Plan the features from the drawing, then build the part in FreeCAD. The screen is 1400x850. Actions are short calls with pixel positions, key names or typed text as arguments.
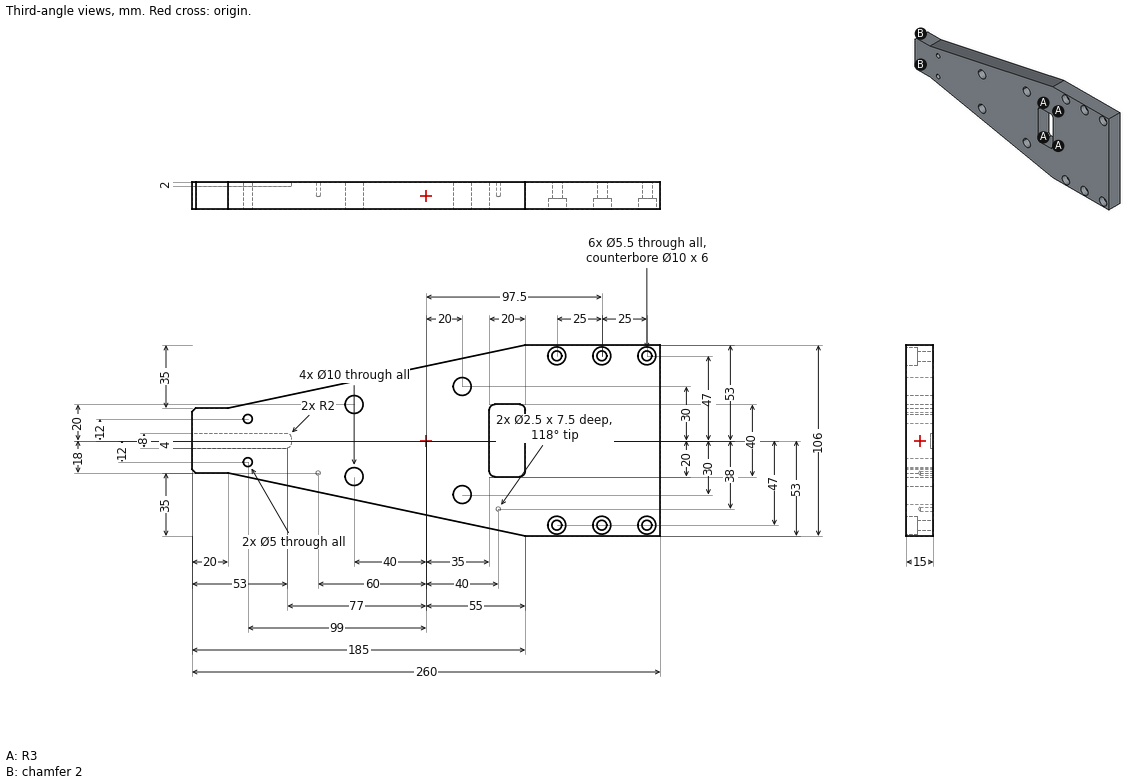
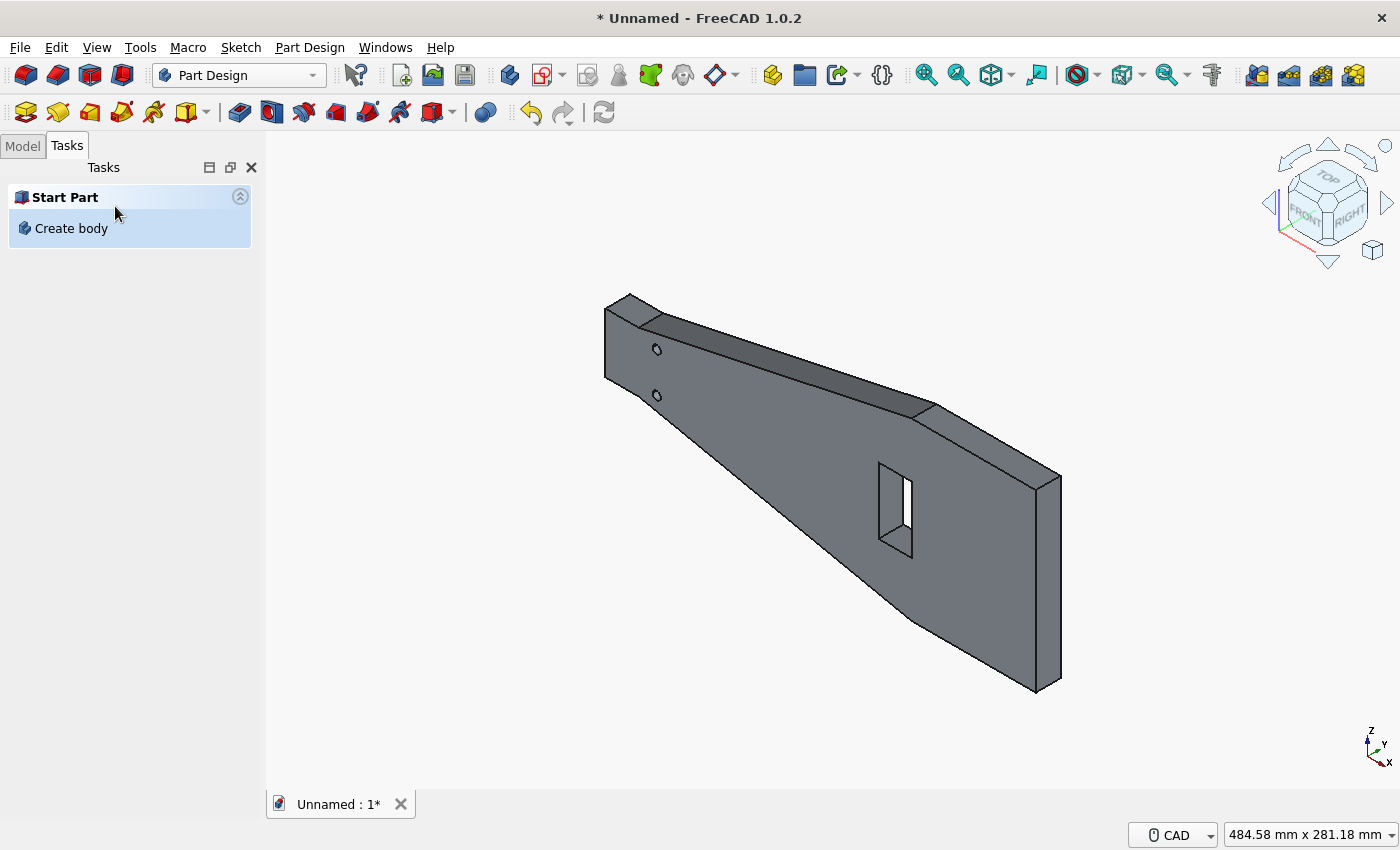
key(2)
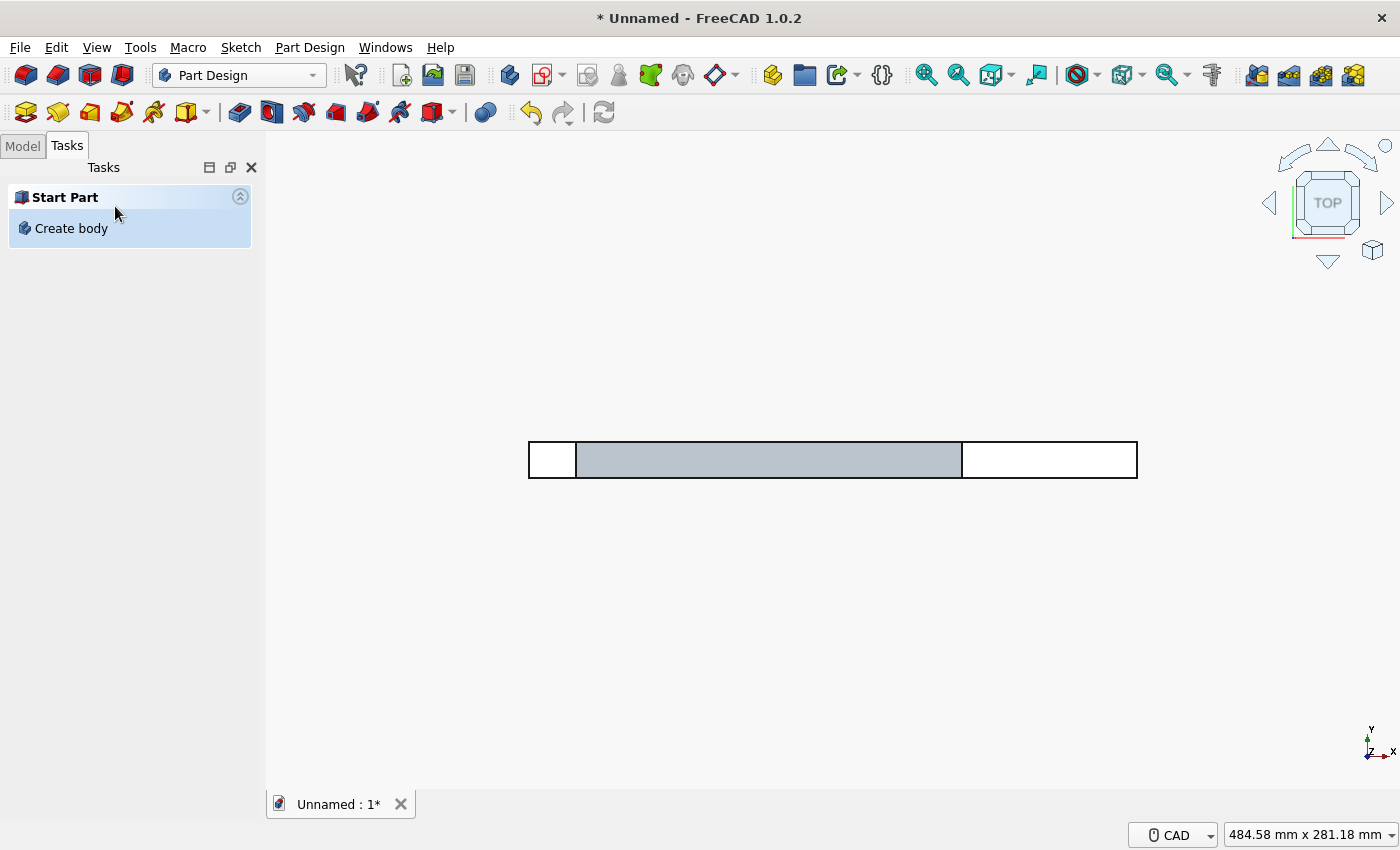
key(1)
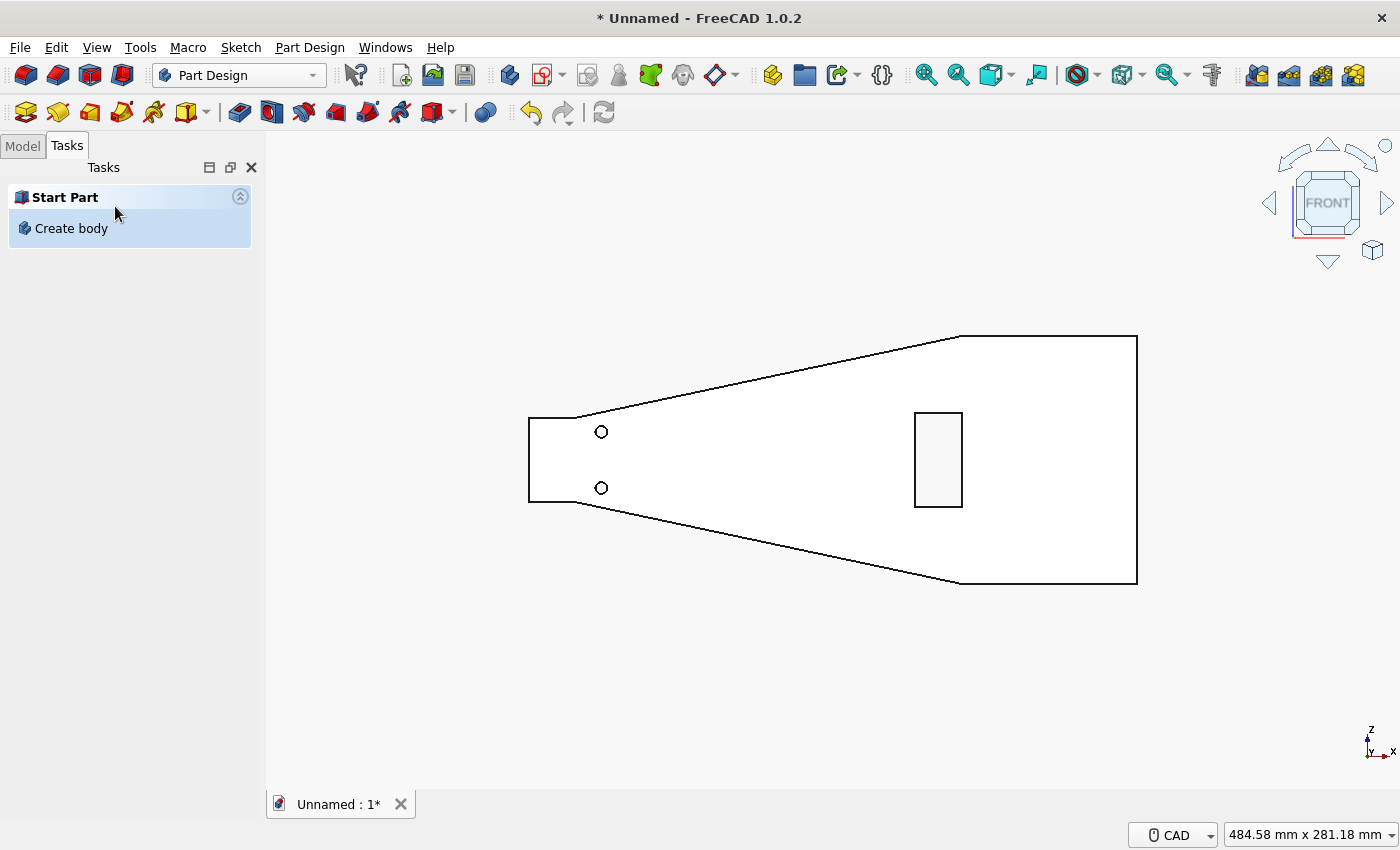
key(3)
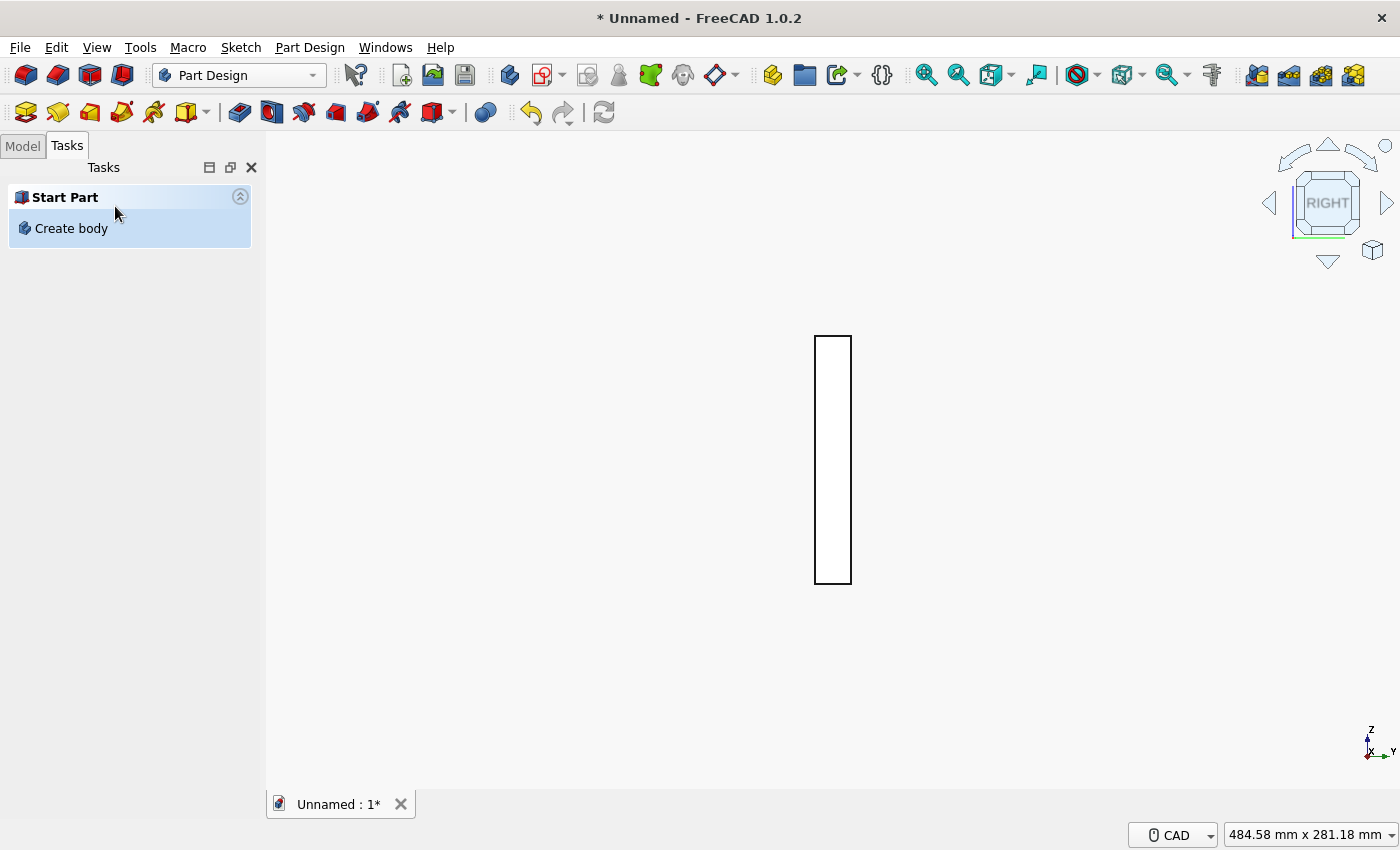
key(v)
key(f)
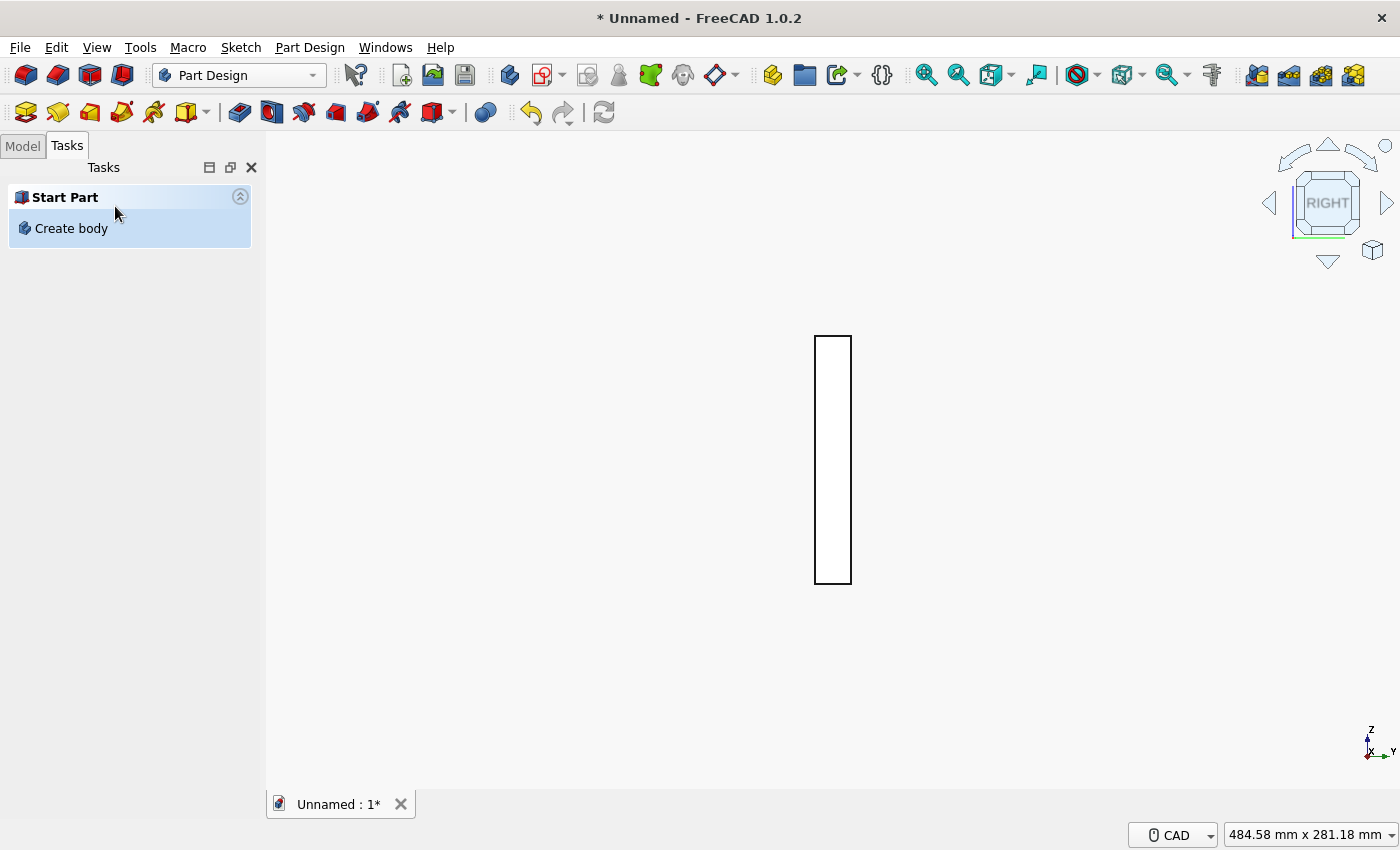
key(5)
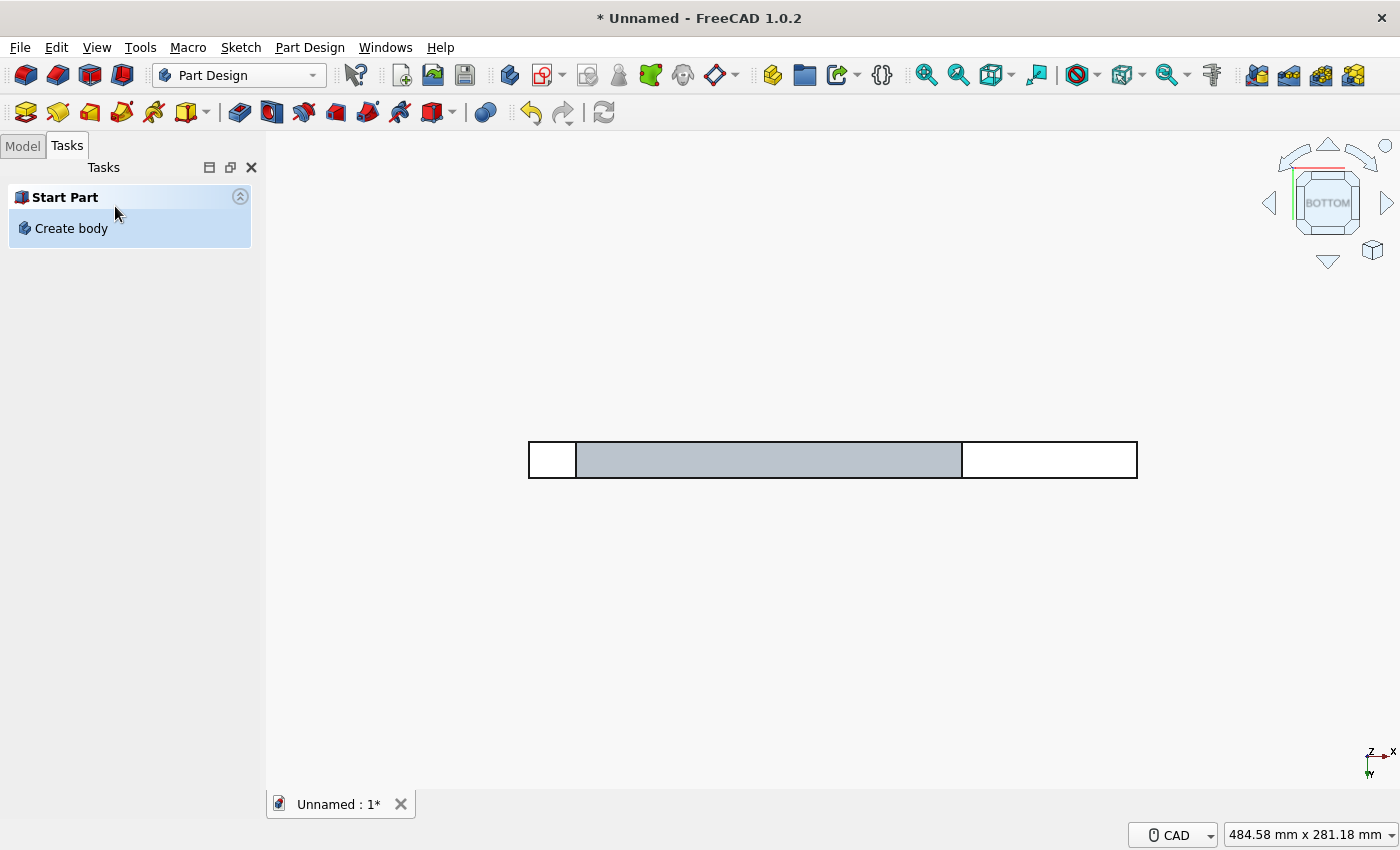
key(4)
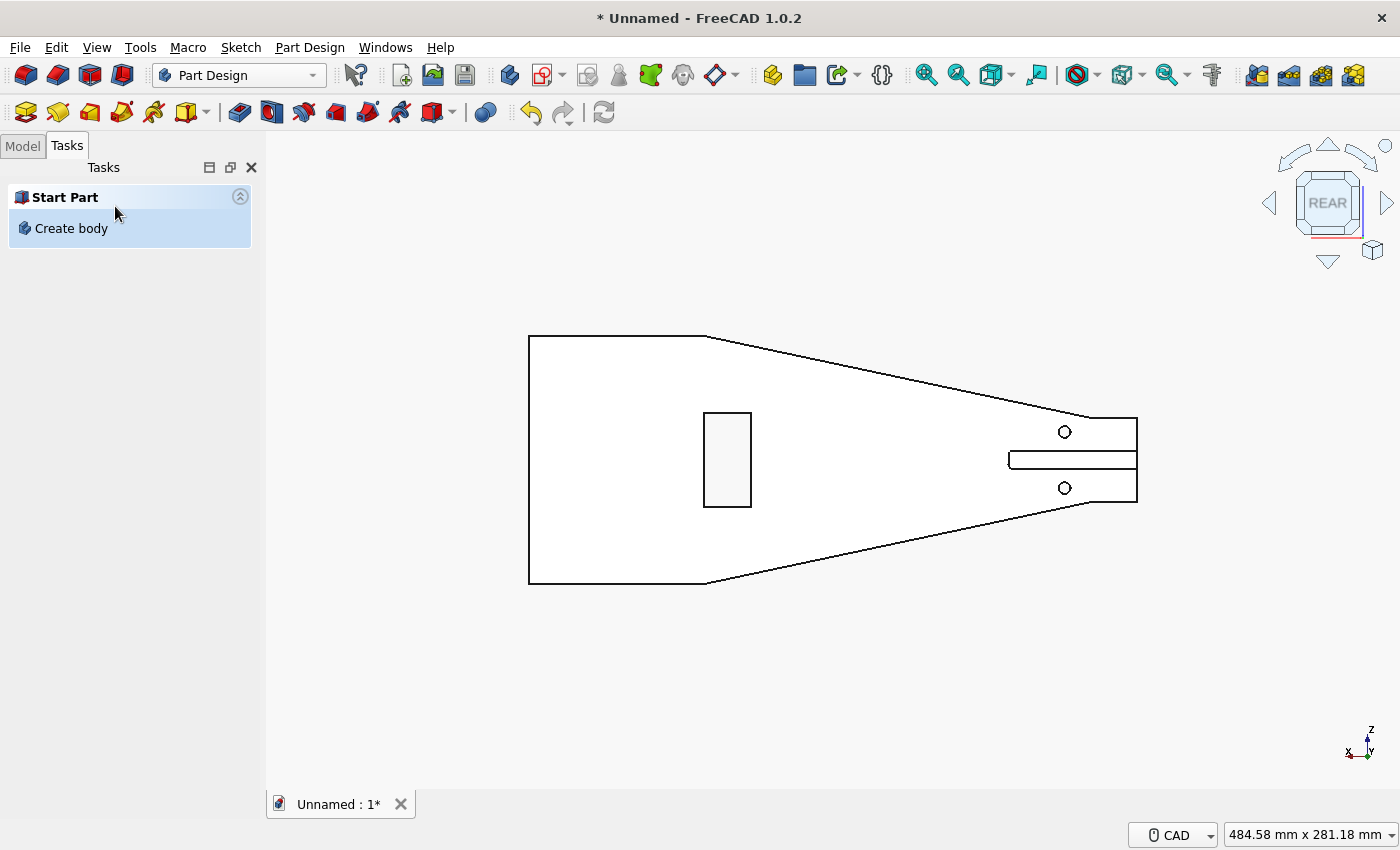
key(6)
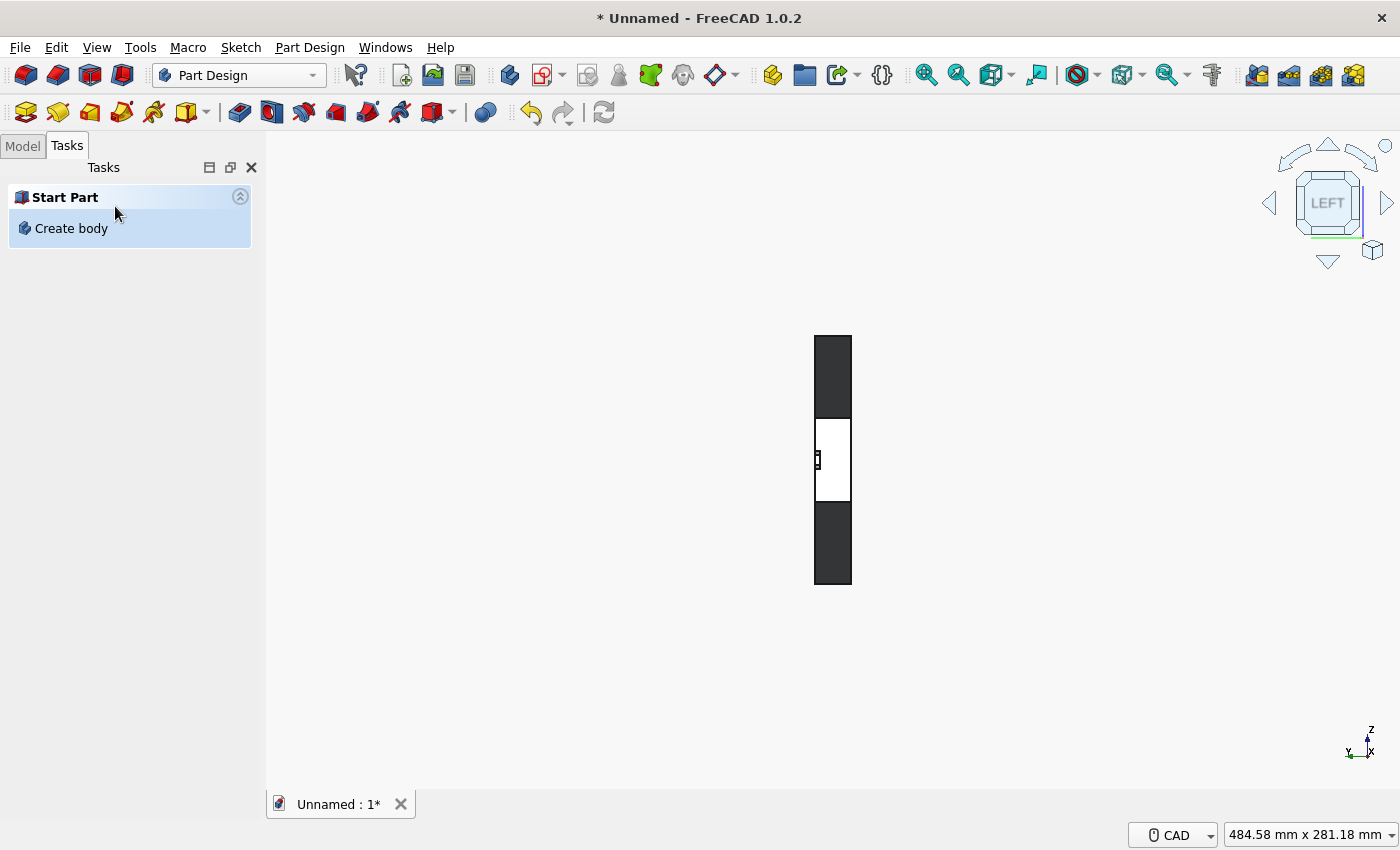
key(v)
key(f)